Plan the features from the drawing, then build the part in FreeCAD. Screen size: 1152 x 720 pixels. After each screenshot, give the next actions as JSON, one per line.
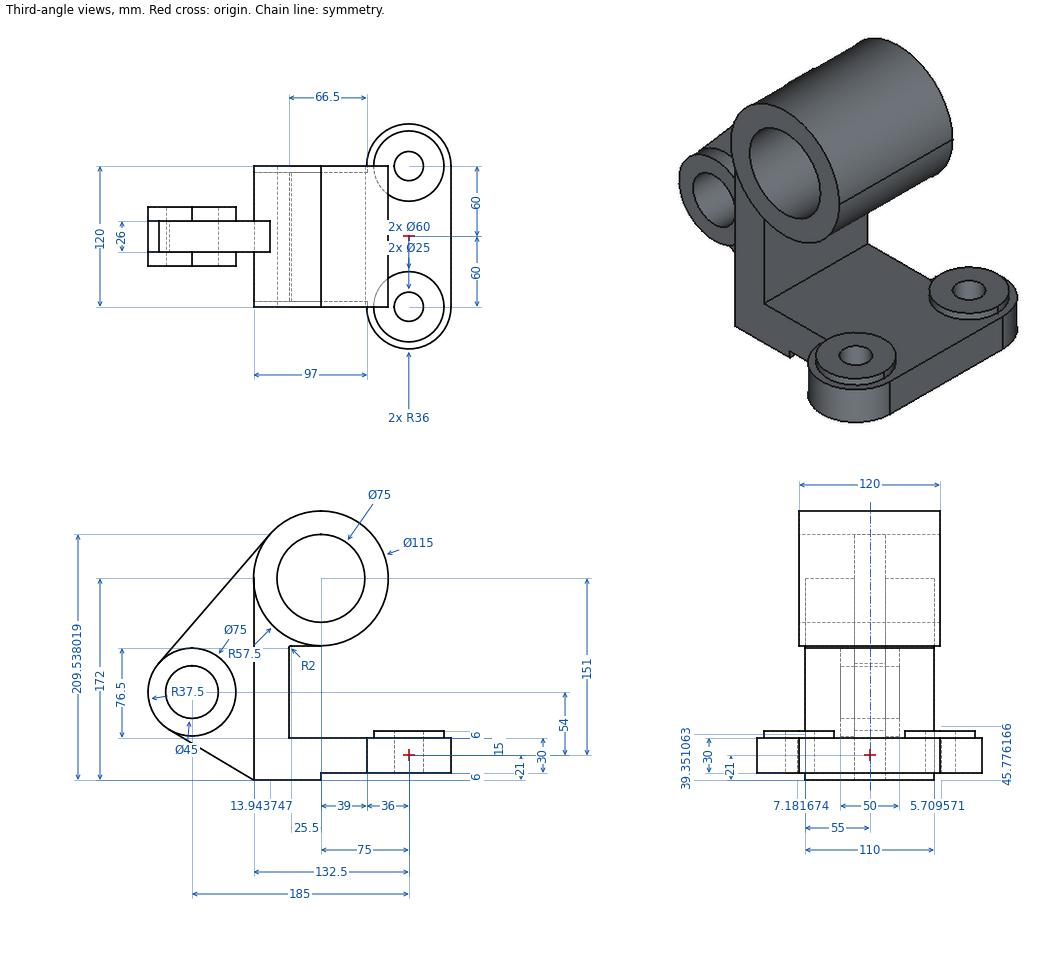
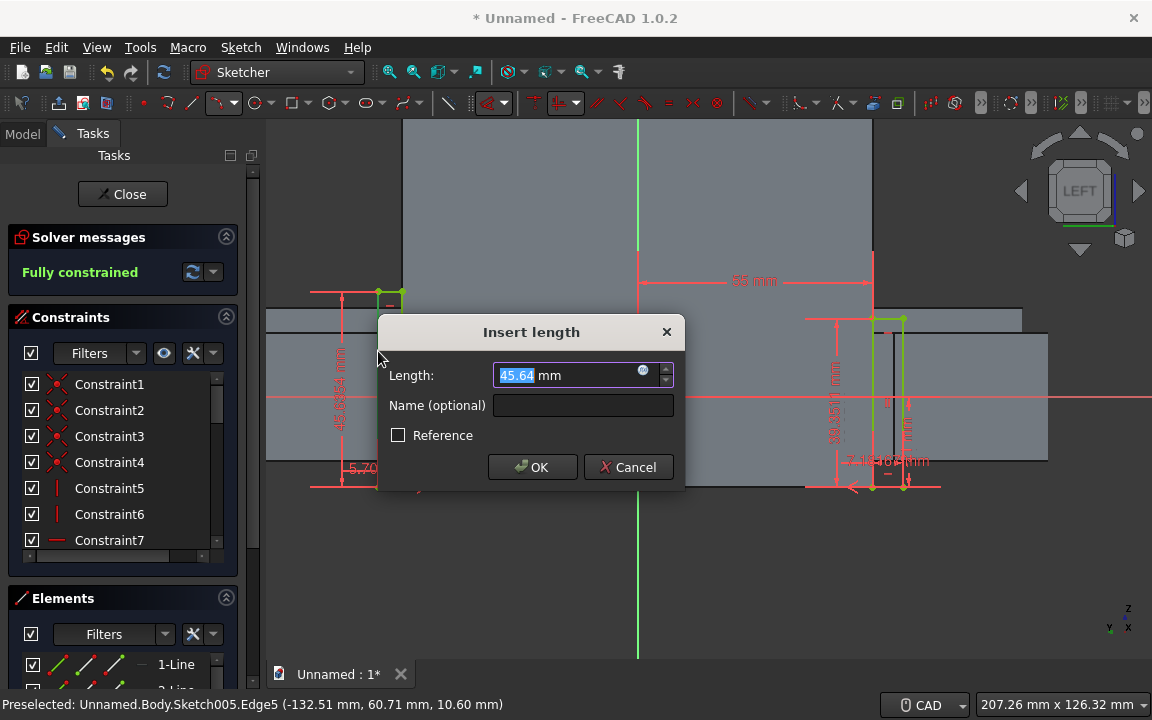
{"action": "type", "text": "45.776166"}
{"action": "key", "text": "Return"}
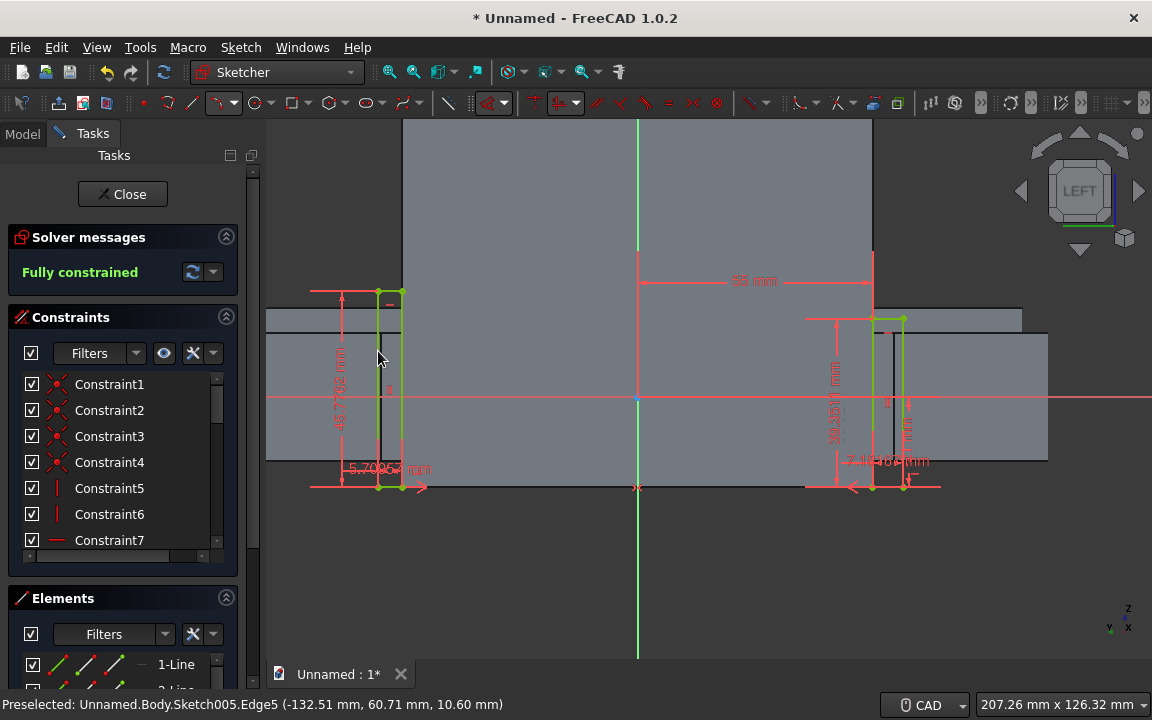
{"action": "left_click", "coordinate": [123, 194]}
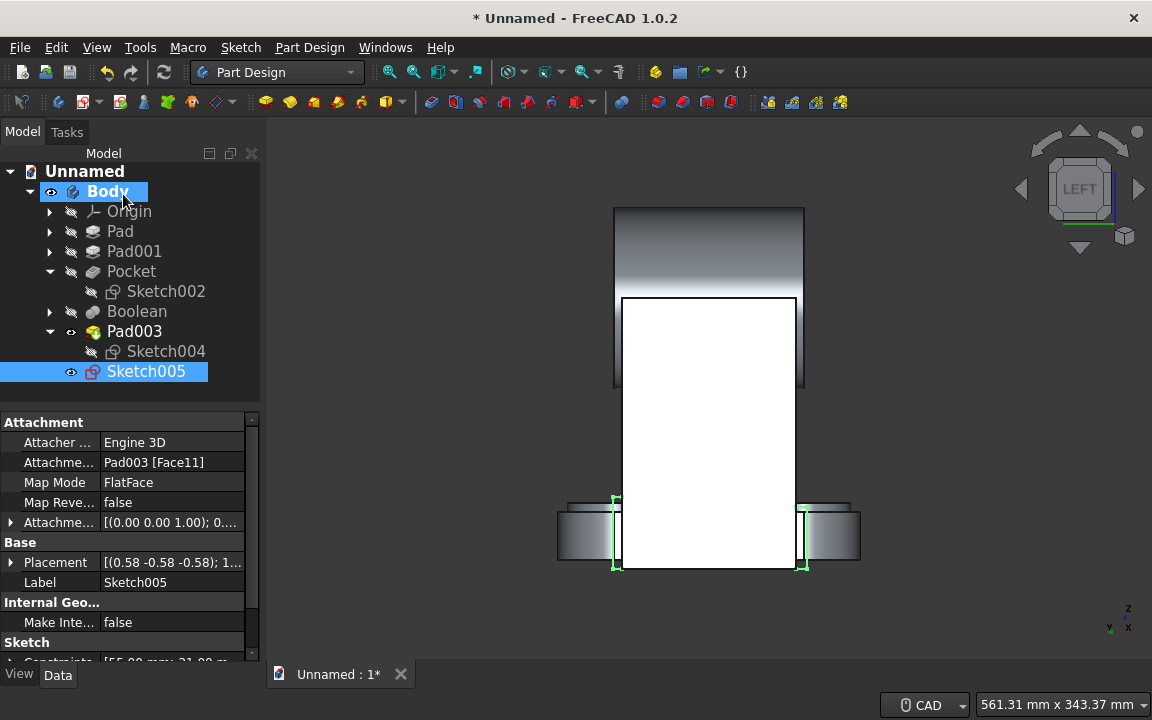
{"action": "left_click", "coordinate": [432, 102]}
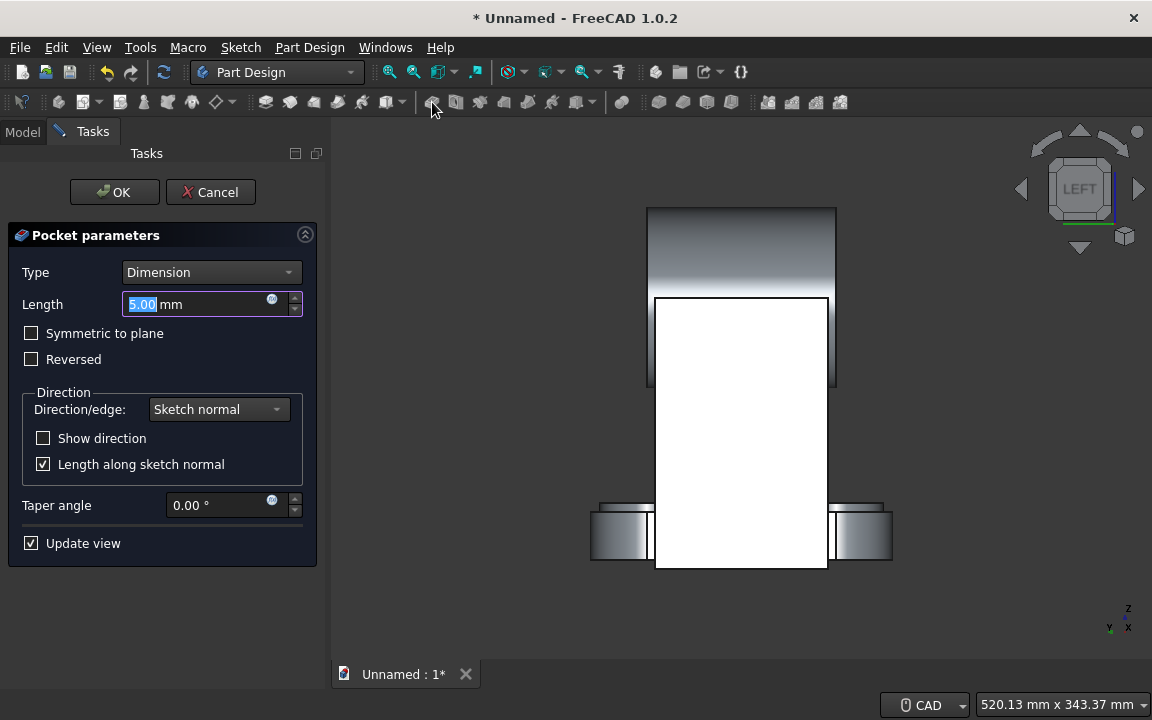
{"action": "type", "text": "97"}
{"action": "key", "text": "Tab"}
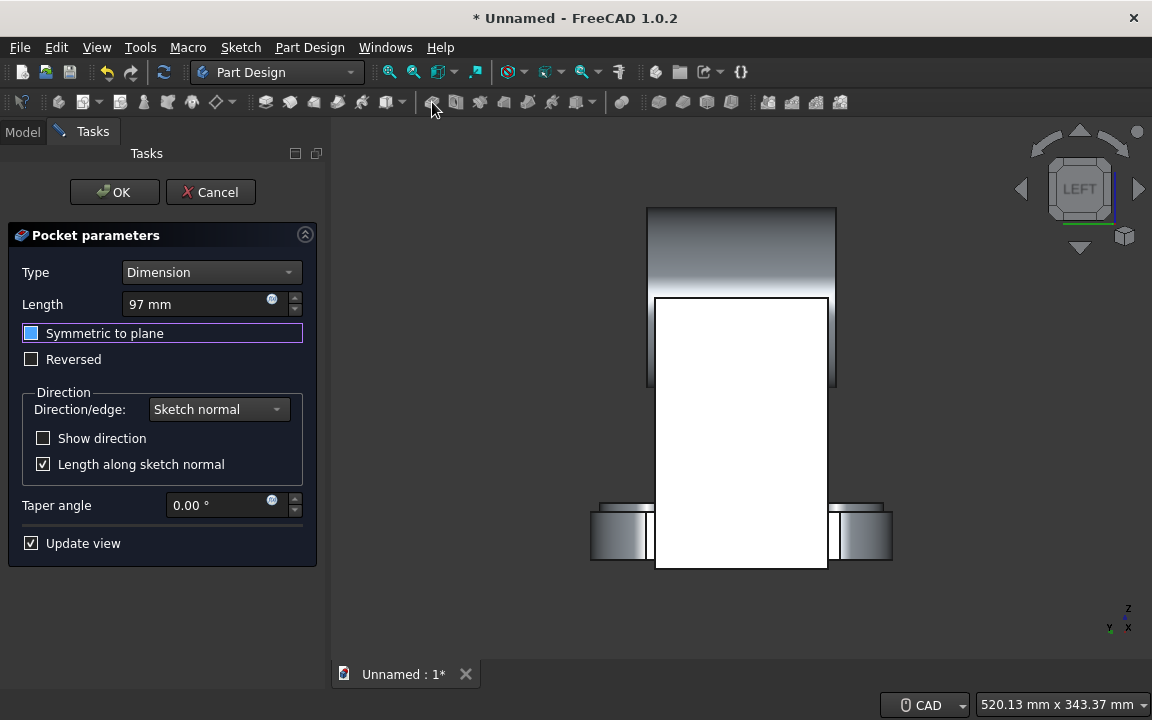
{"action": "left_click", "coordinate": [115, 192]}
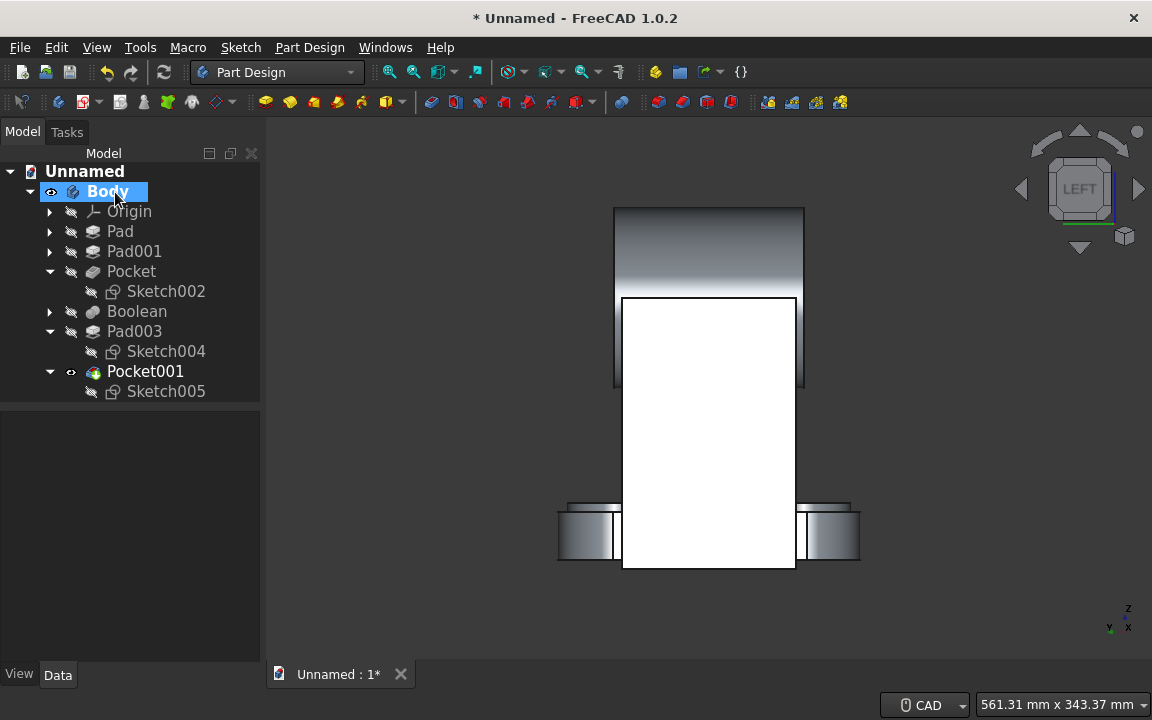
{"action": "left_click", "coordinate": [60, 102]}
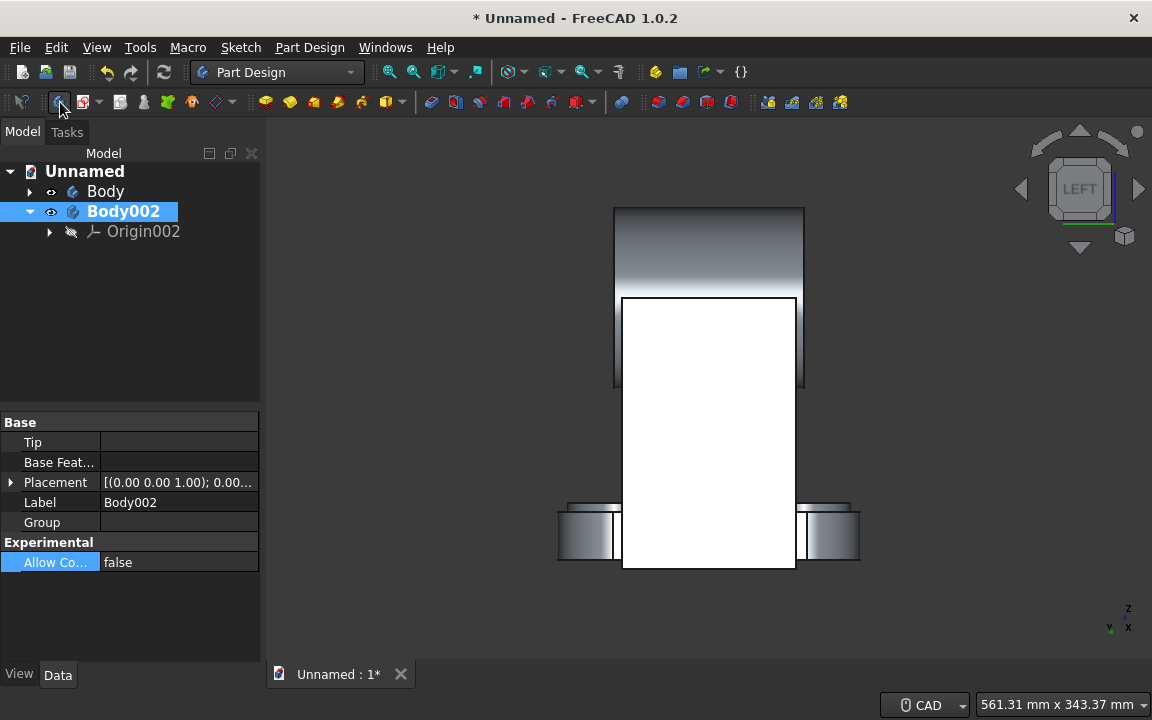
{"action": "left_click", "coordinate": [306, 619]}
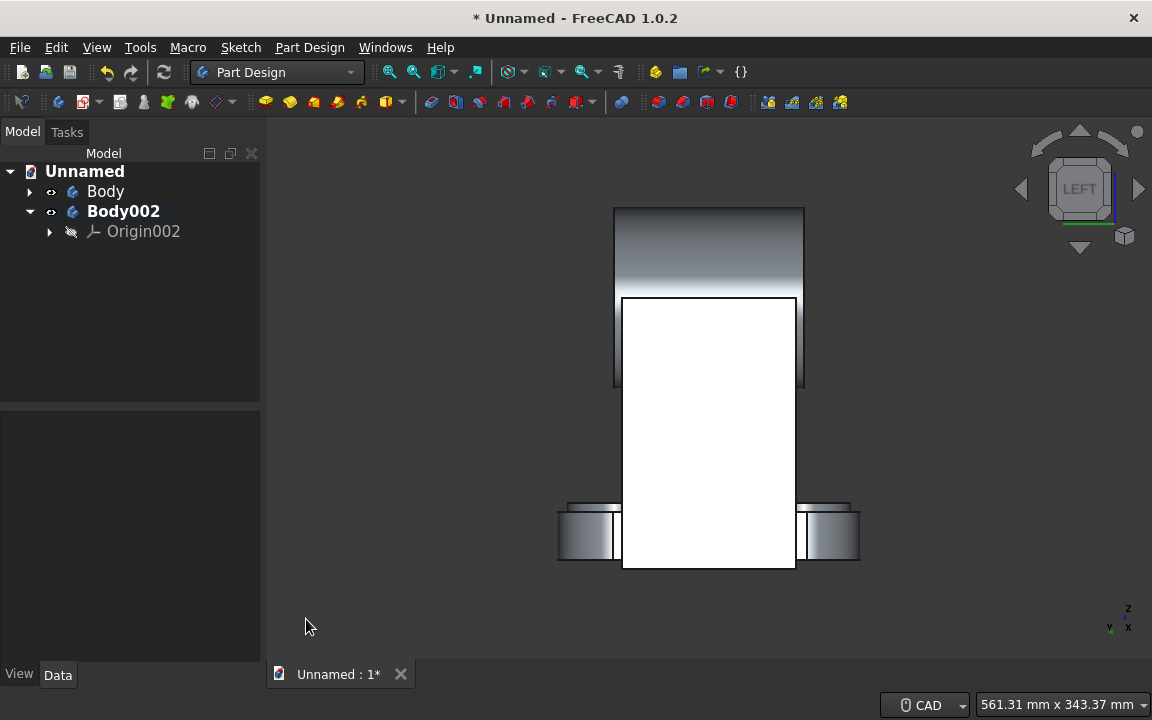
{"action": "left_click", "coordinate": [84, 102]}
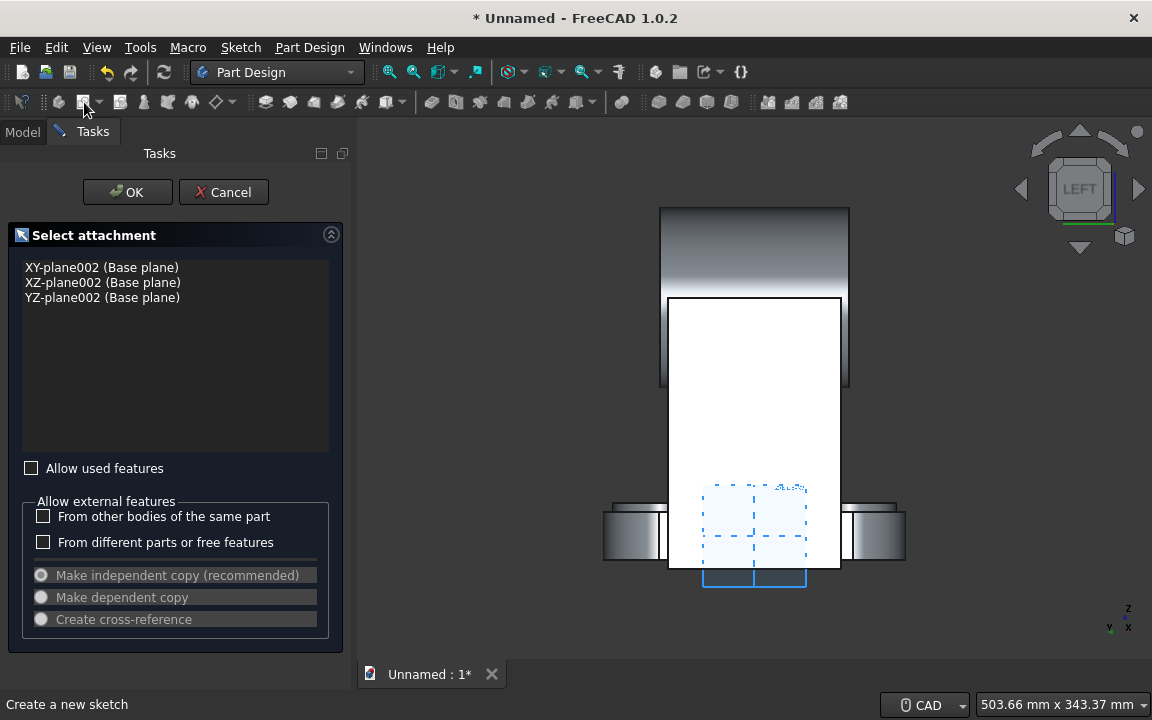
{"action": "left_click", "coordinate": [82, 282]}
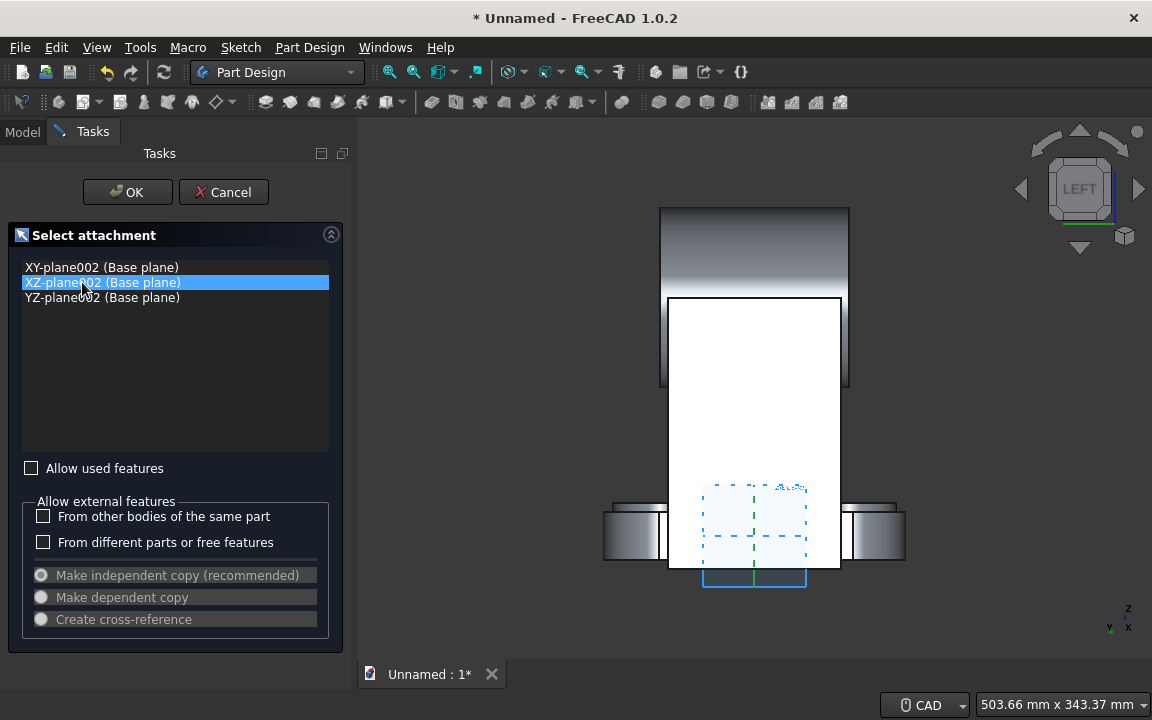
{"action": "left_click", "coordinate": [128, 192]}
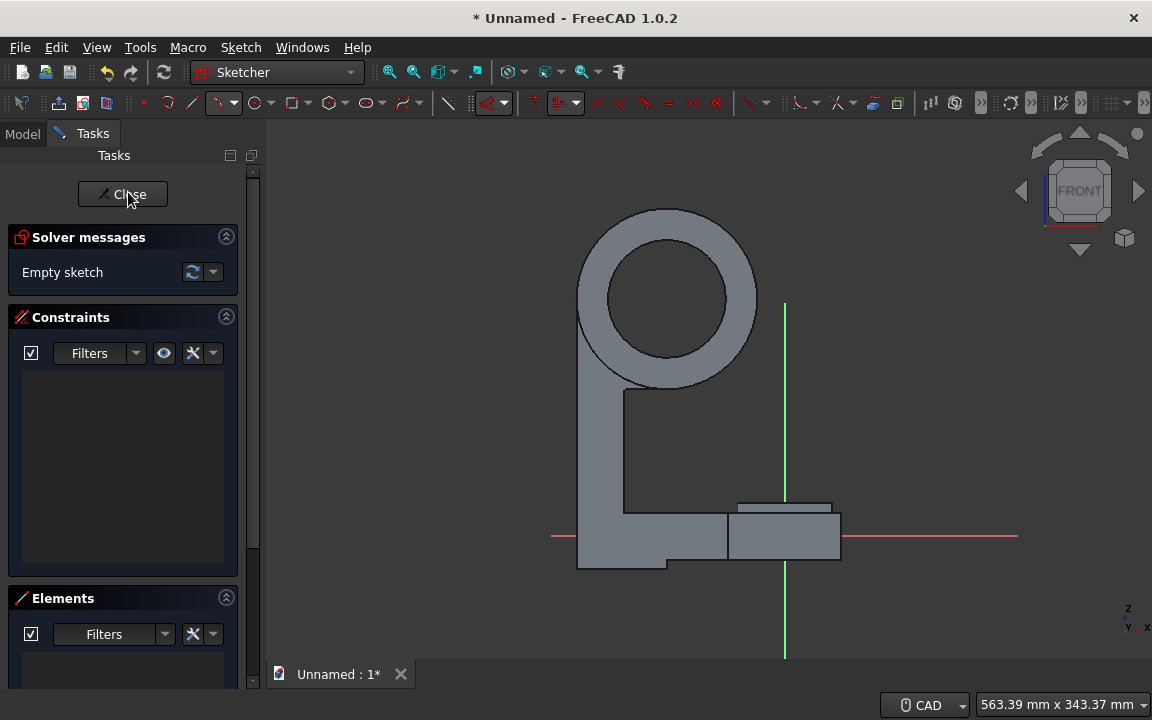
{"action": "scroll", "coordinate": [409, 488], "scroll_direction": "up", "scroll_amount": 5}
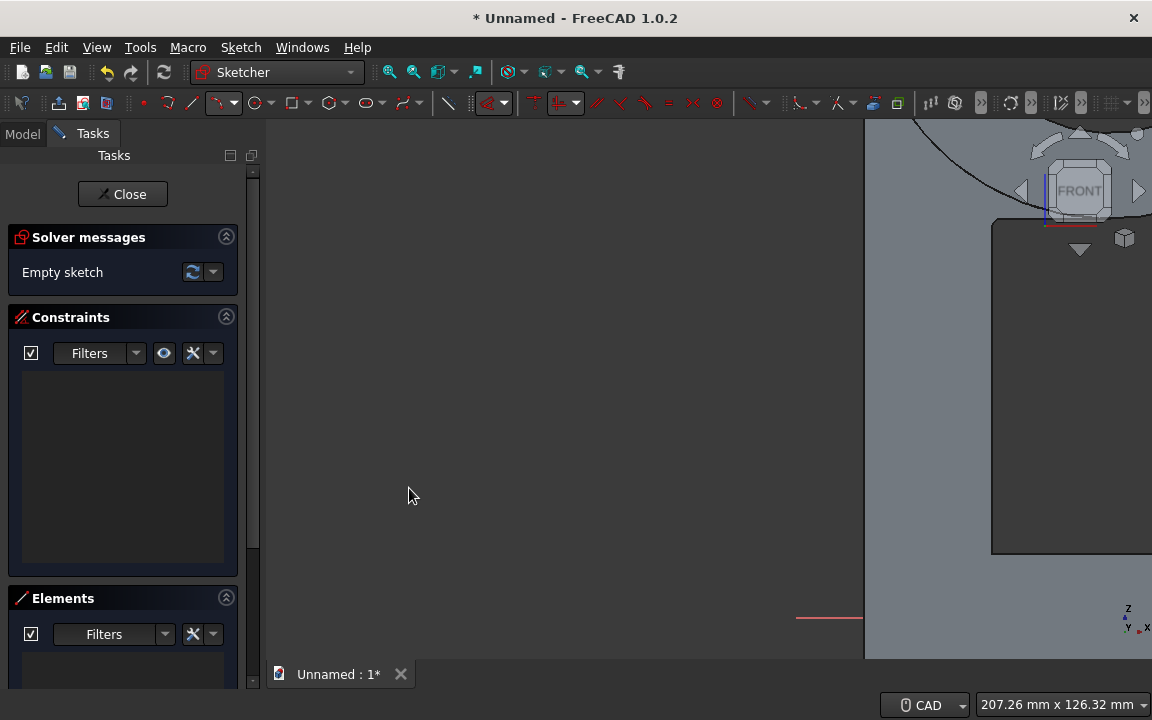
{"action": "left_click", "coordinate": [256, 104]}